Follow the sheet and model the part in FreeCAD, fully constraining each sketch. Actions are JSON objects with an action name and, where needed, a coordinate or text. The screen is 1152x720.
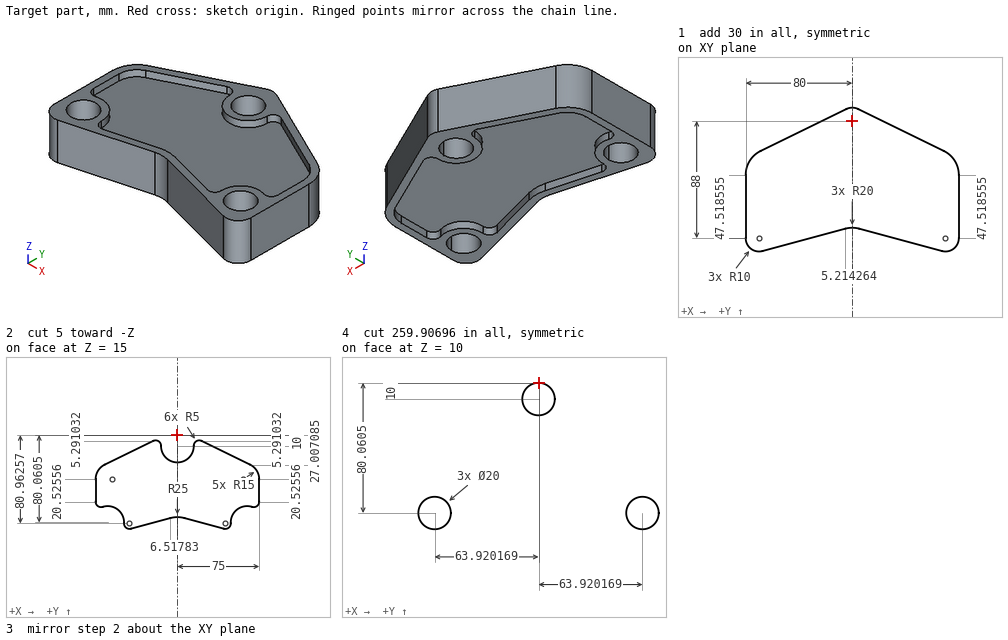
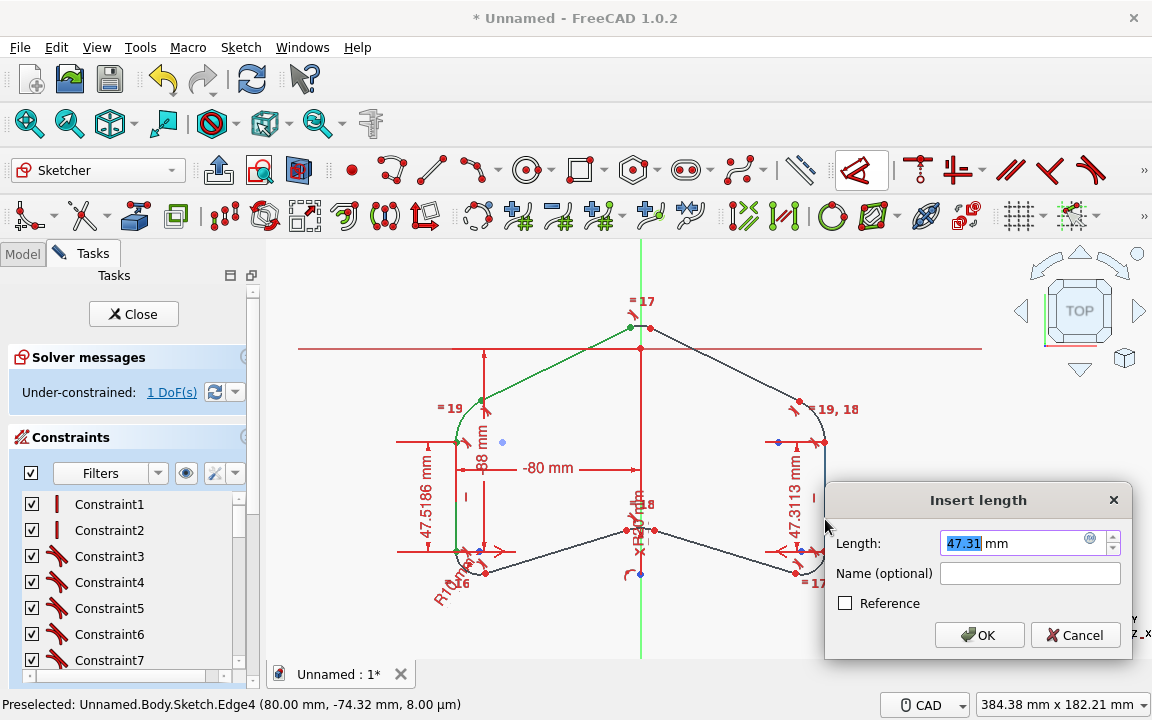
{"action": "type", "text": "47.518555"}
{"action": "key", "text": "Return"}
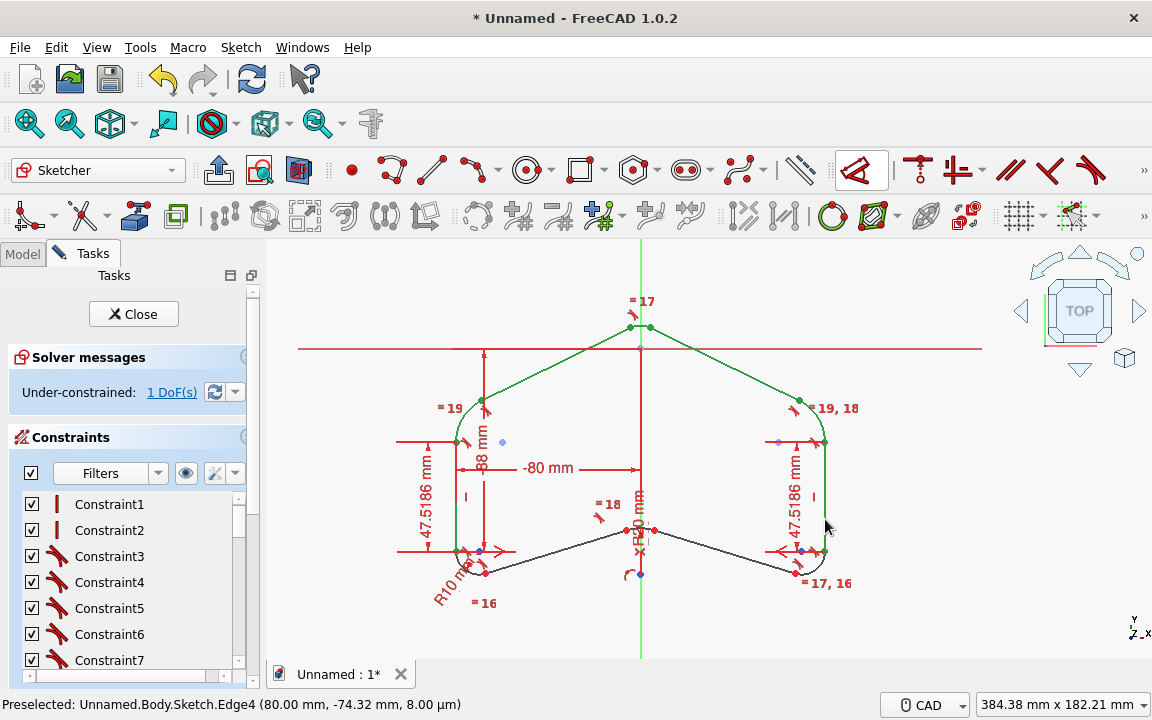
{"action": "scroll", "coordinate": [627, 530], "scroll_direction": "up", "scroll_amount": 6}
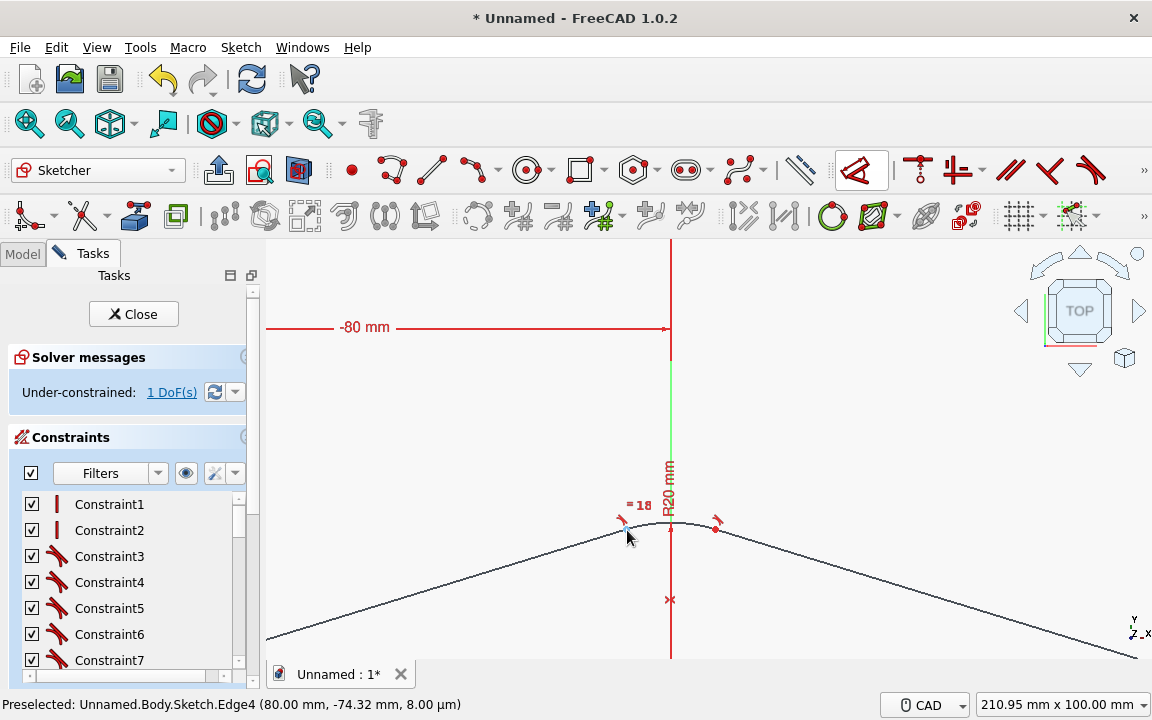
{"action": "left_click", "coordinate": [626, 529]}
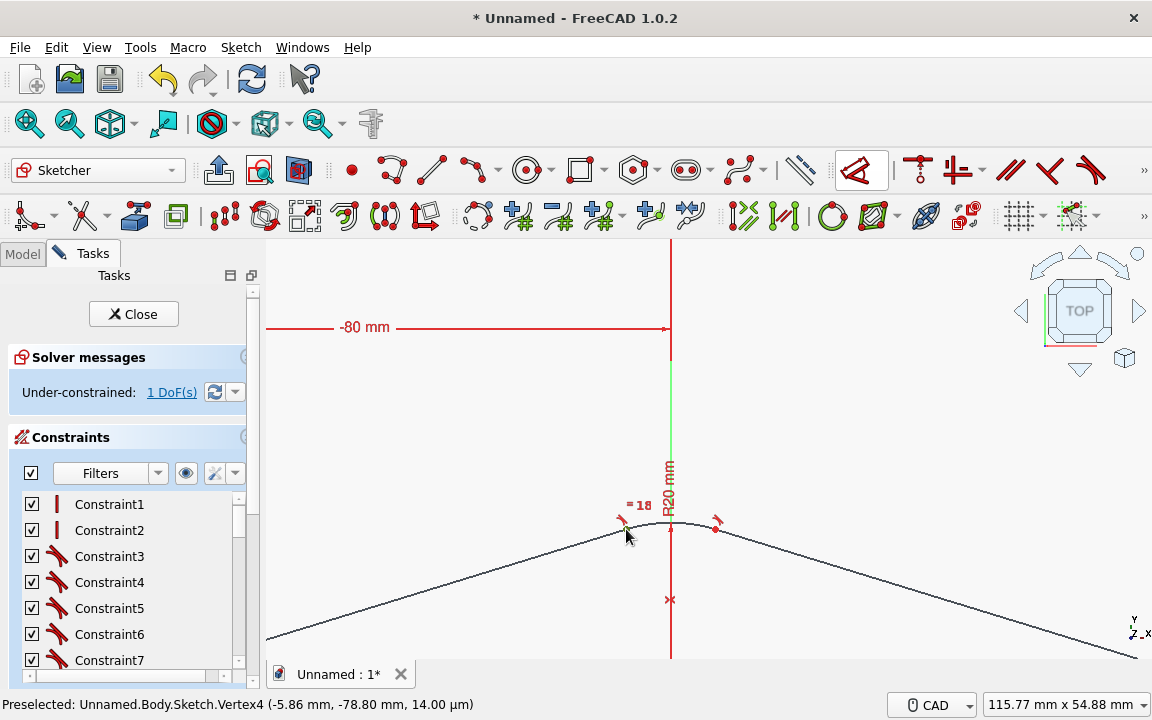
{"action": "left_click", "coordinate": [882, 170]}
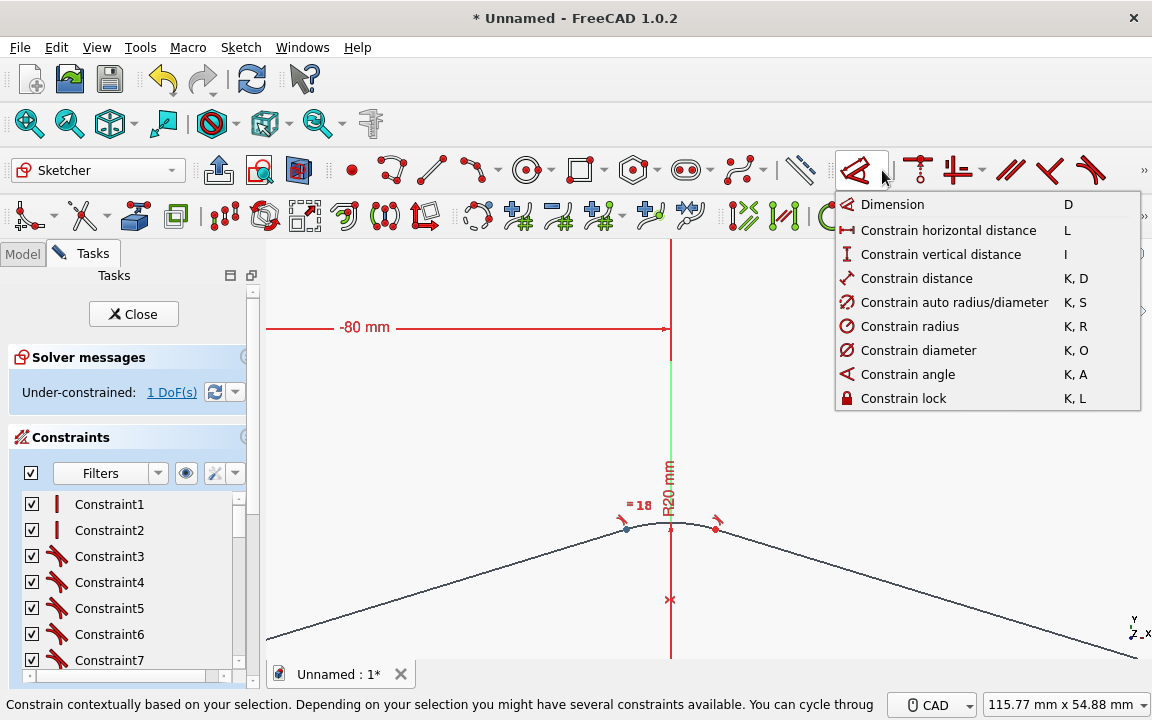
{"action": "left_click", "coordinate": [988, 230]}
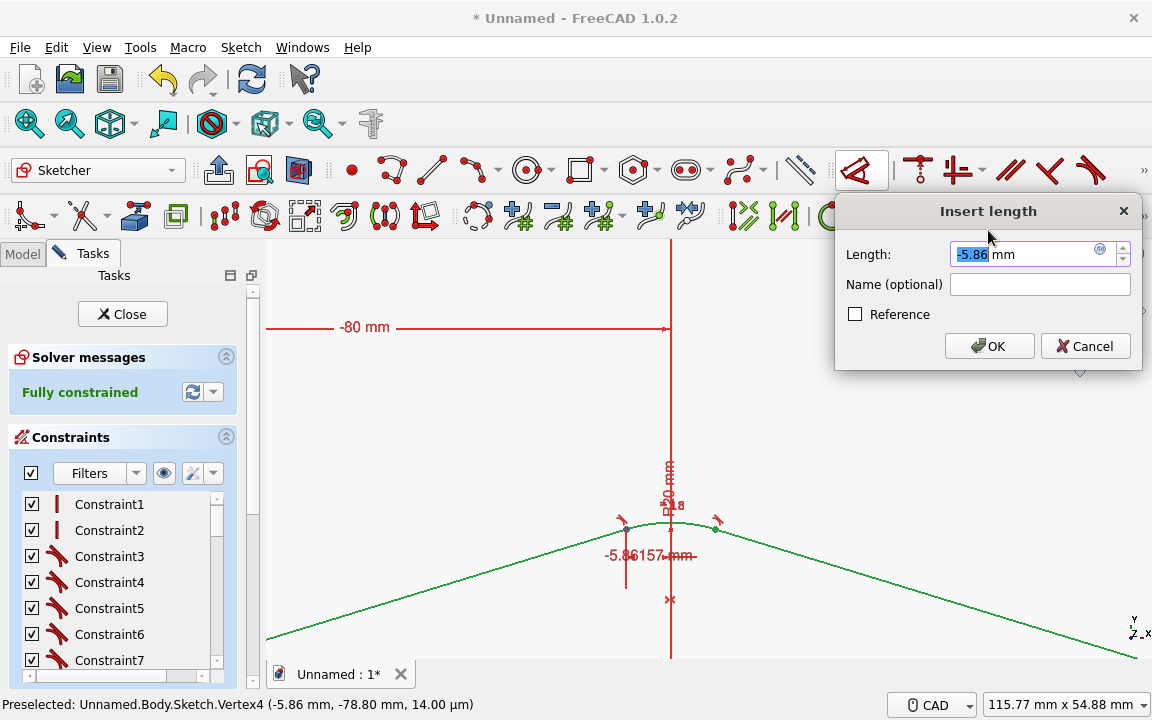
{"action": "type", "text": "-5.214264"}
{"action": "key", "text": "Return"}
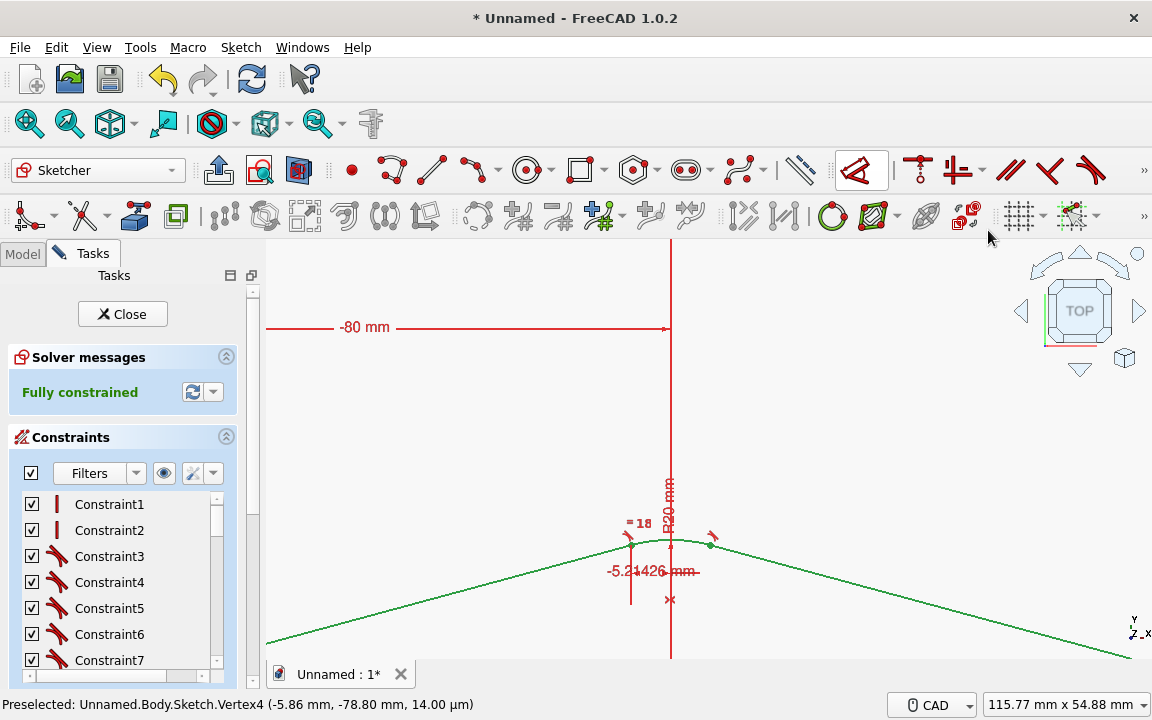
{"action": "left_click", "coordinate": [123, 314]}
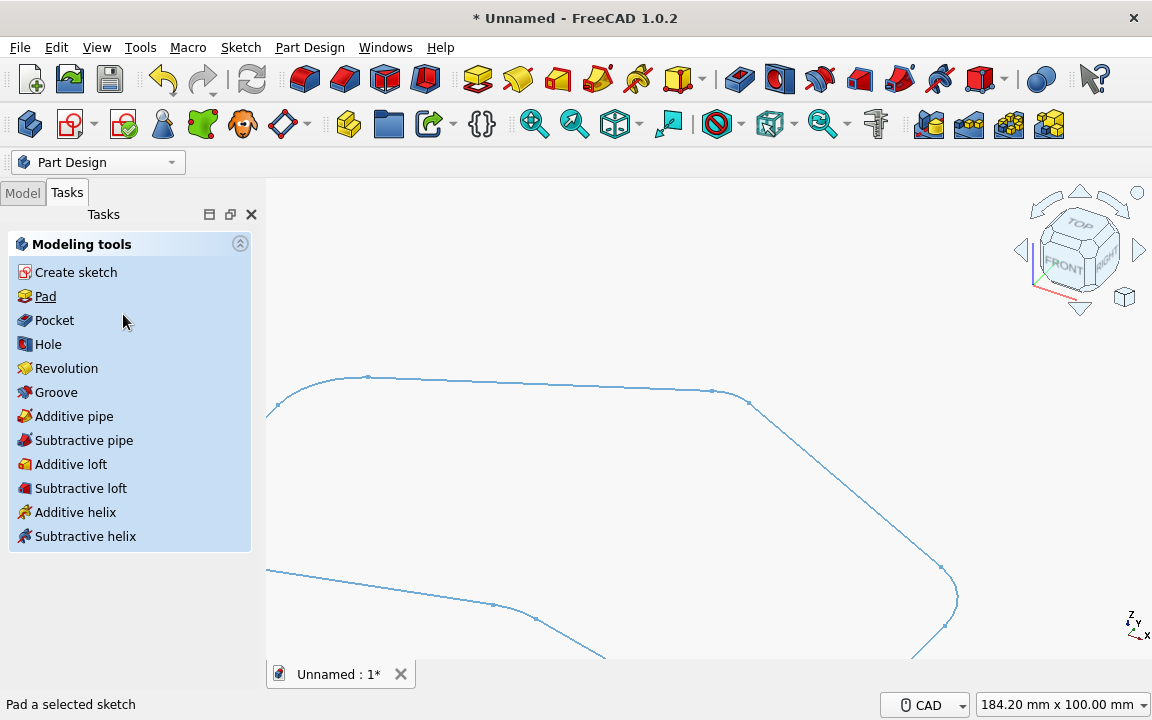
{"action": "left_click", "coordinate": [478, 80]}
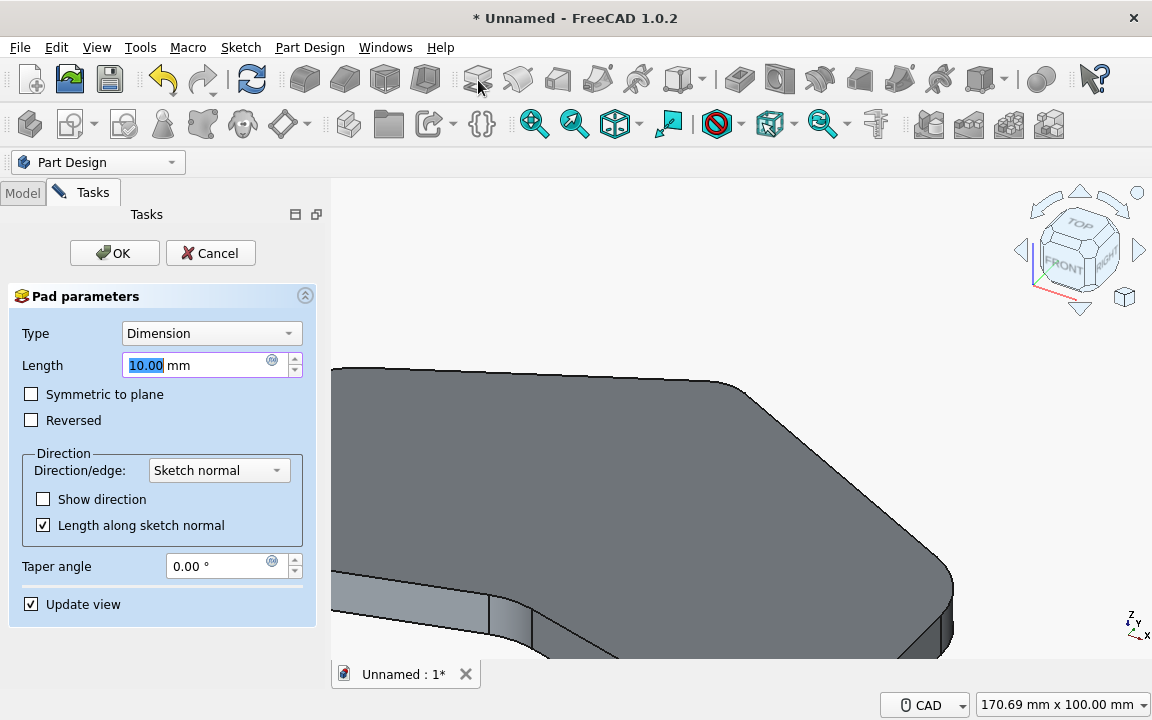
{"action": "type", "text": "30"}
{"action": "key", "text": "Tab"}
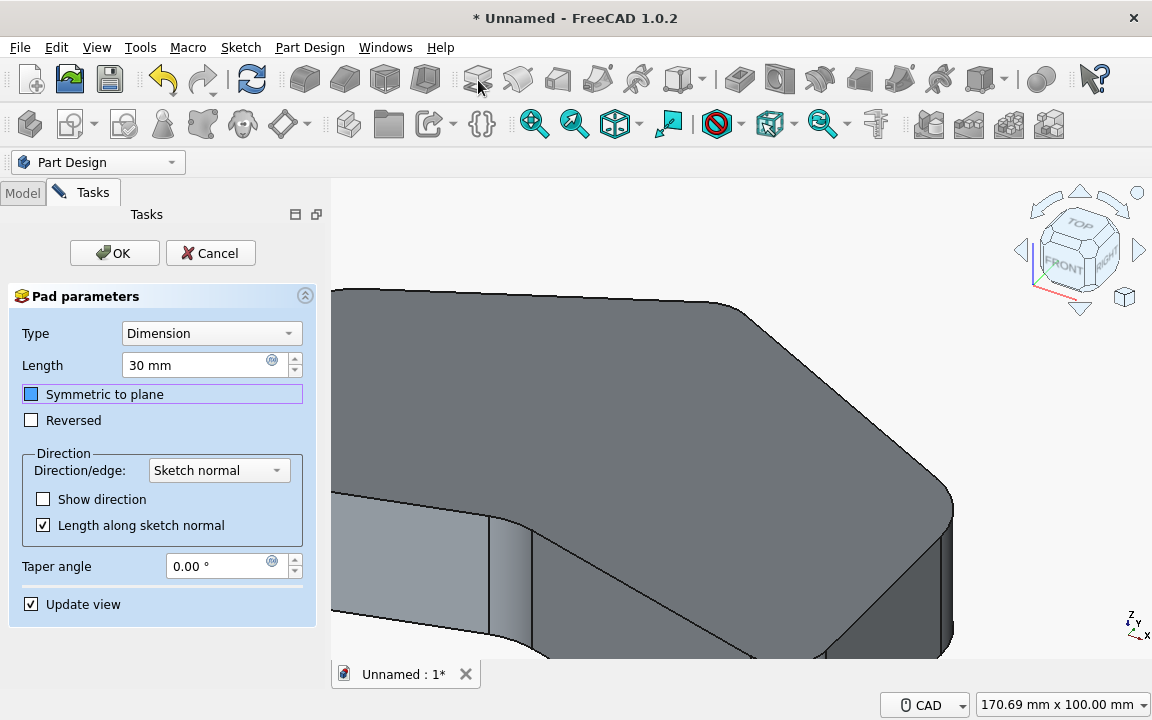
{"action": "left_click", "coordinate": [30, 394]}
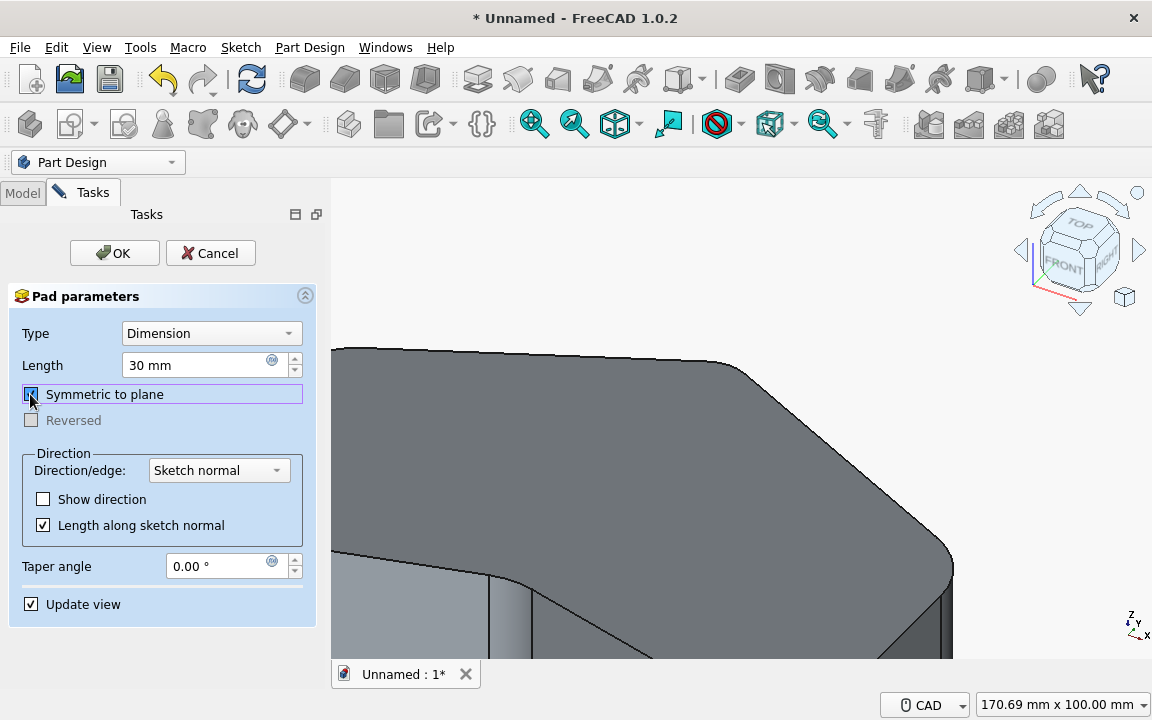
{"action": "left_click", "coordinate": [115, 253]}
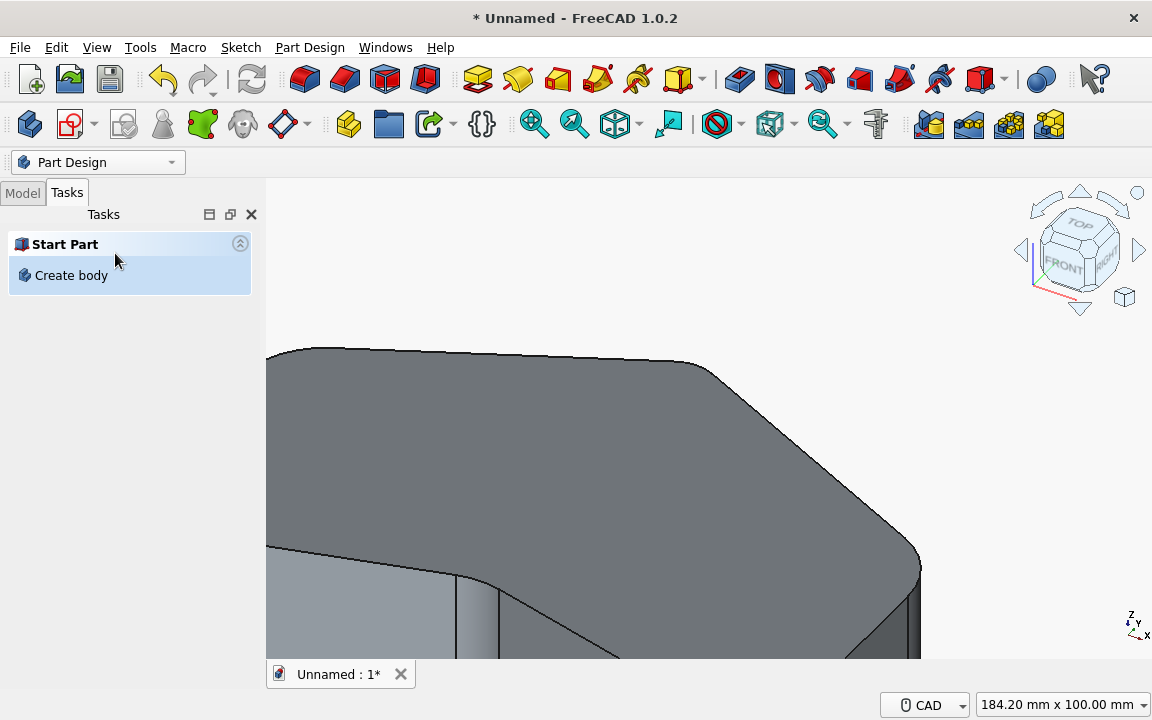
{"action": "key", "text": "v f"}